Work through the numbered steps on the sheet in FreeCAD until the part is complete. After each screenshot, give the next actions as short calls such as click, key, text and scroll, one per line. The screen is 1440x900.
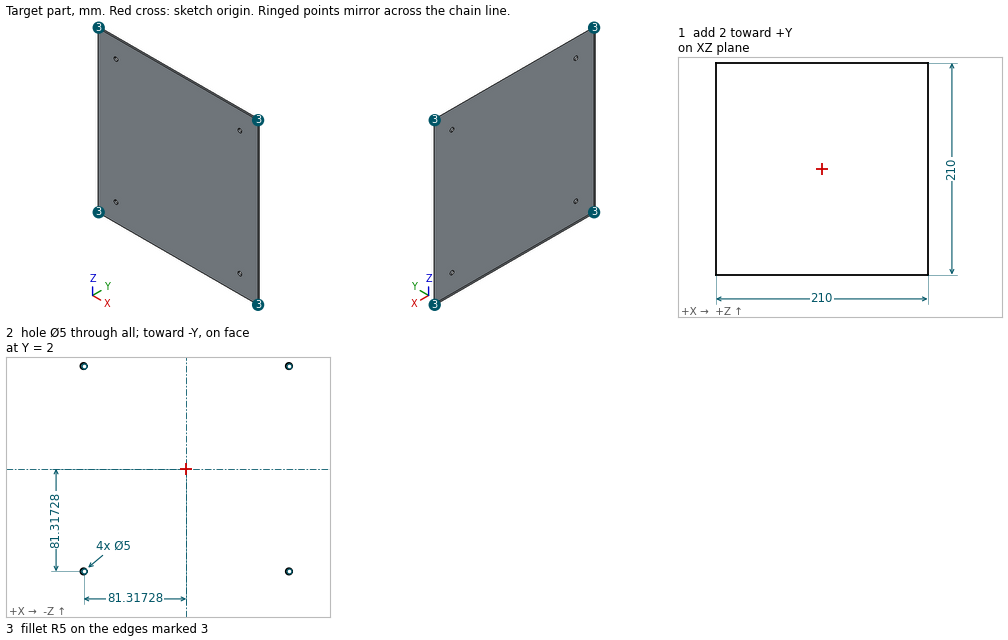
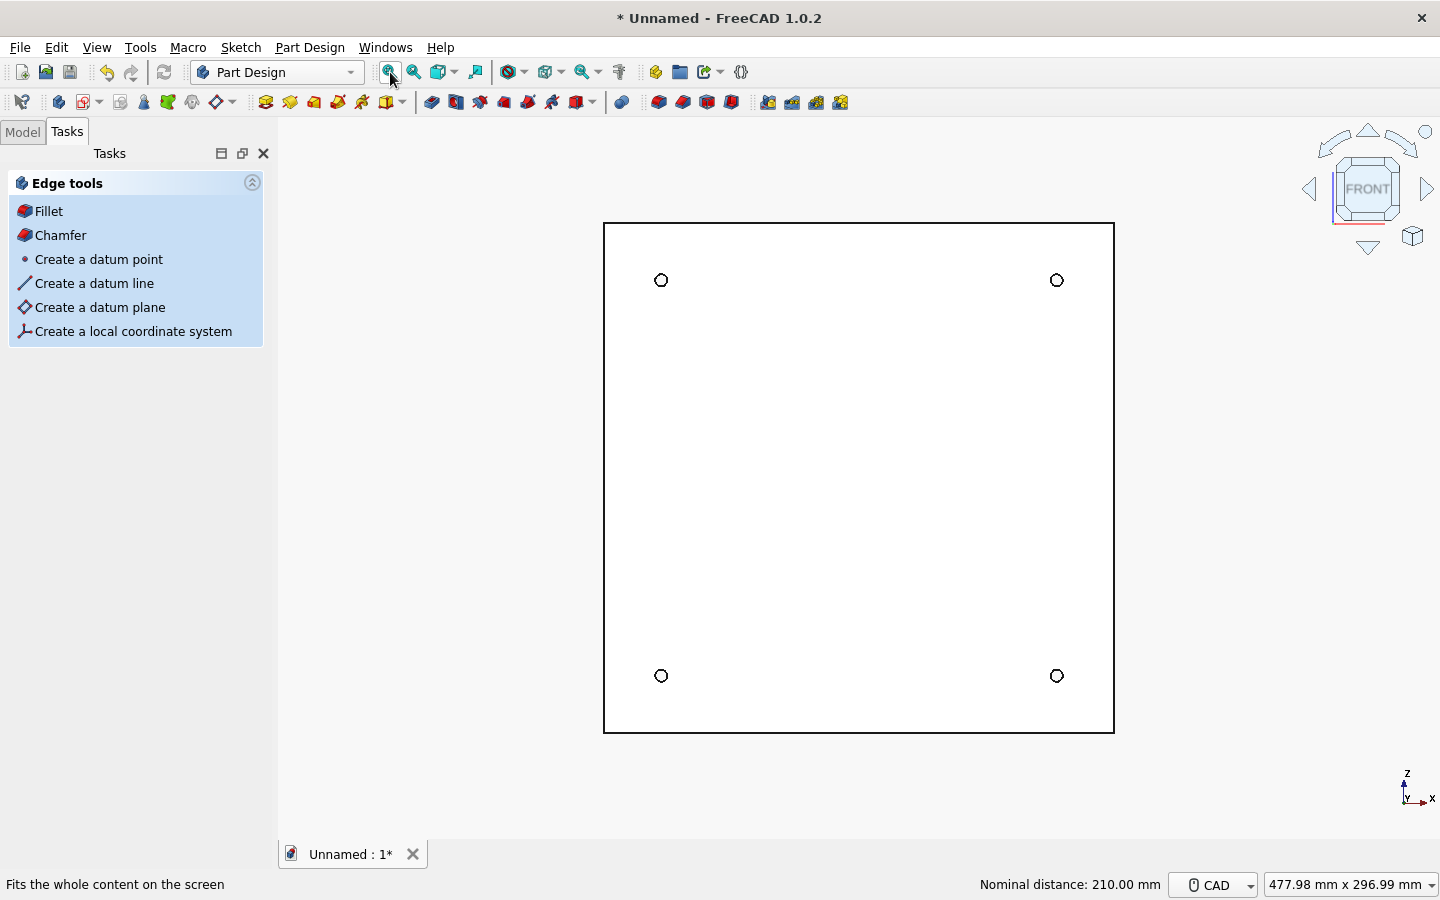
key(3)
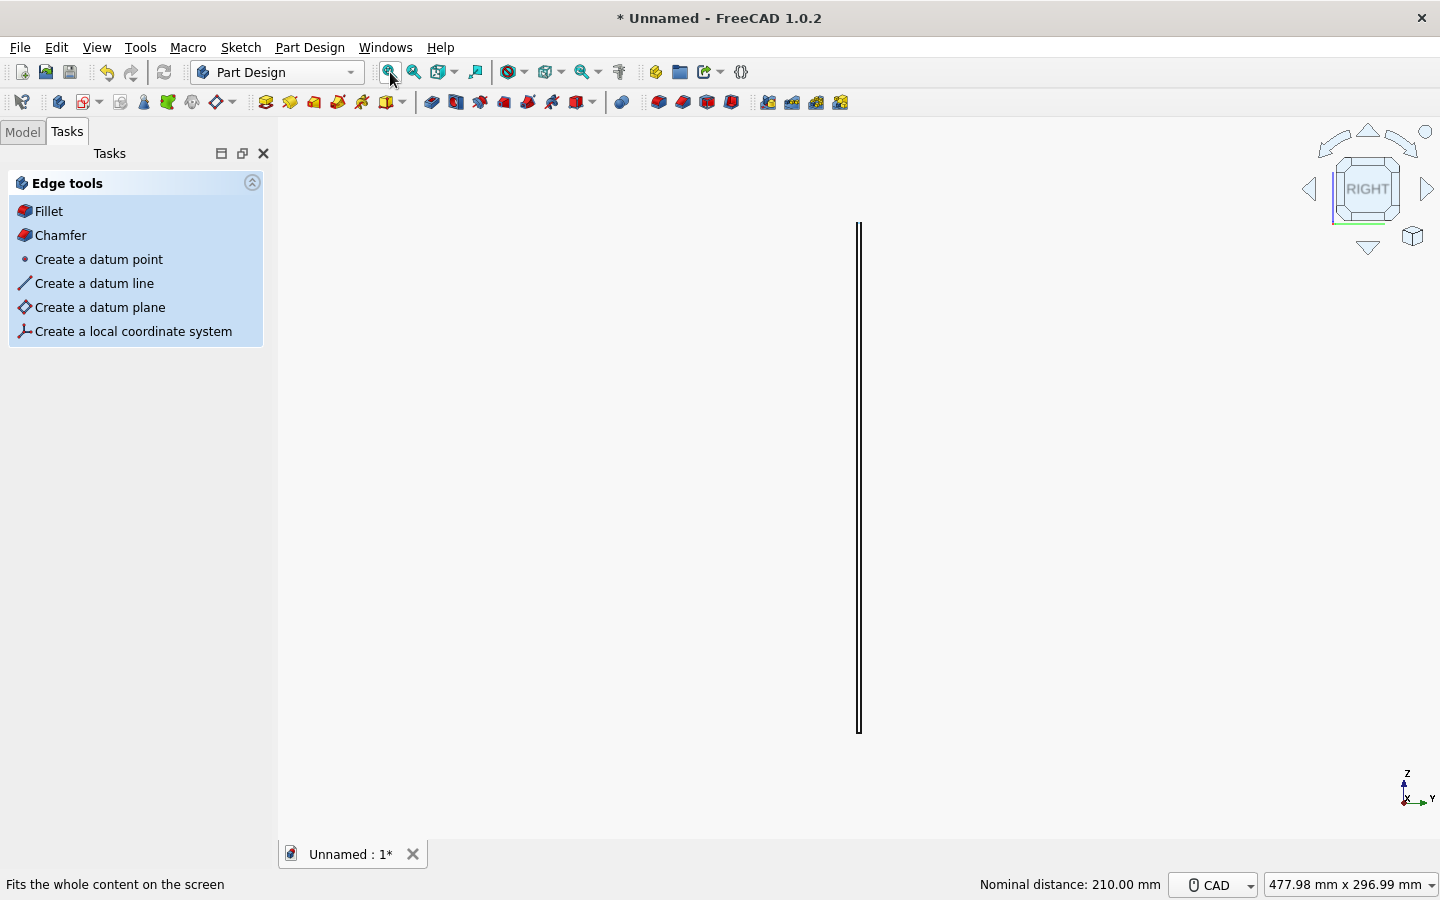
scroll(859, 732, up, 11)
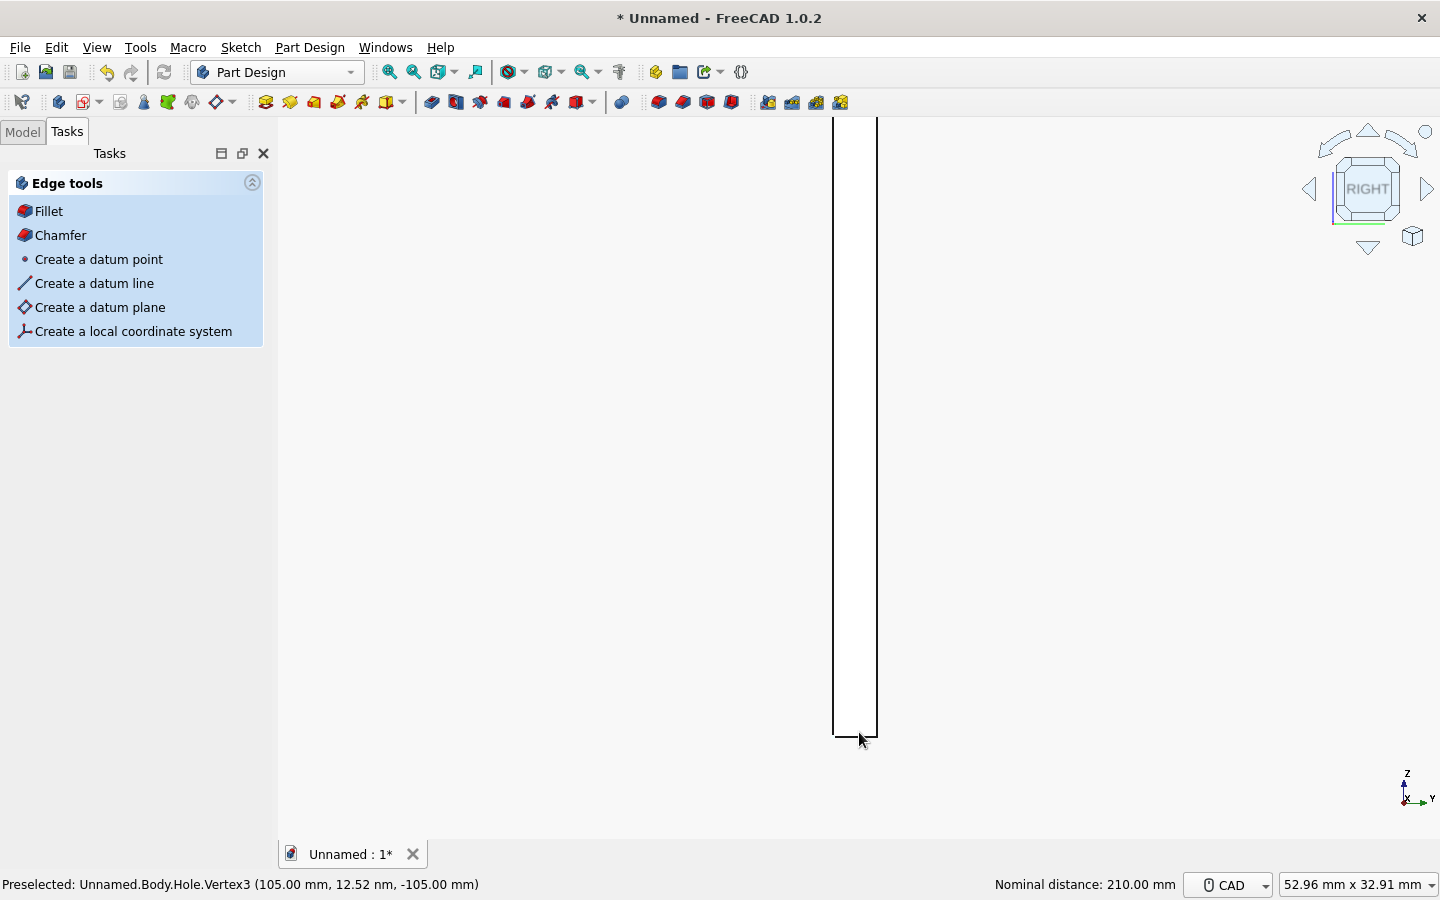
click(855, 736, ctrl)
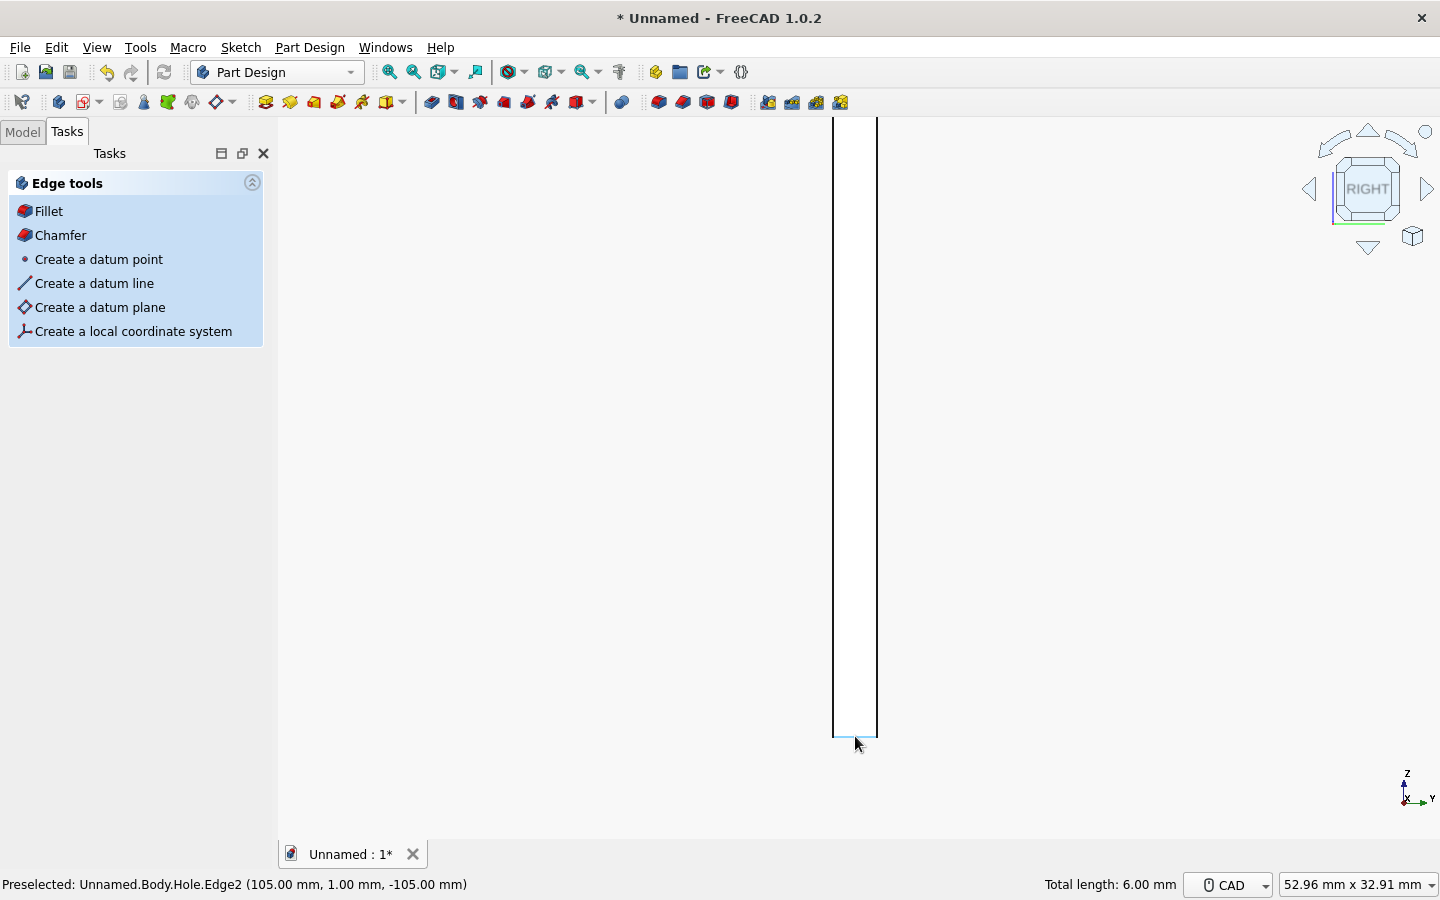
click(390, 72)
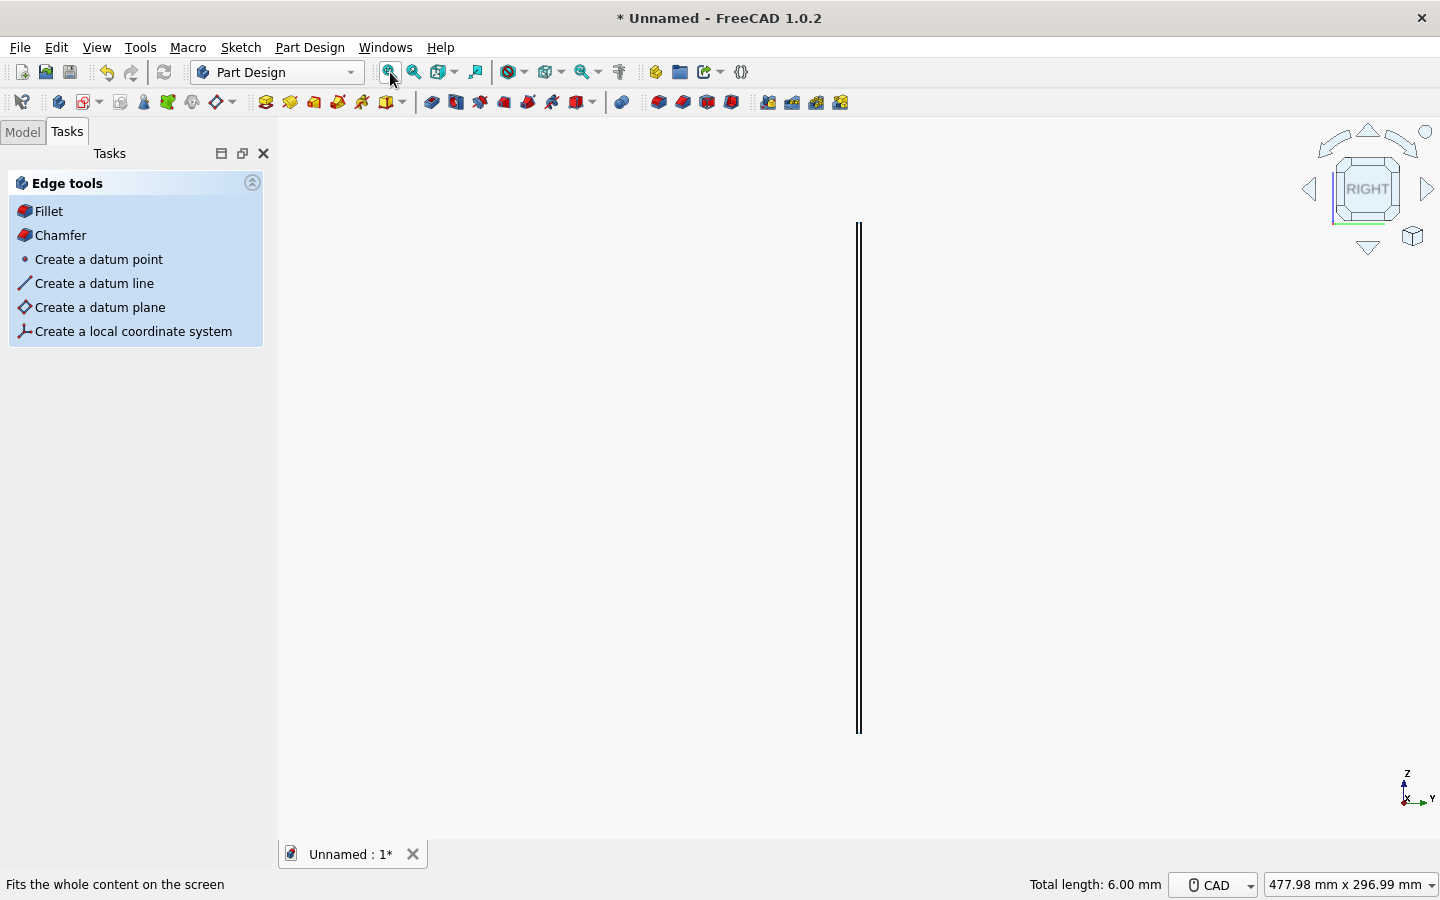
key(5)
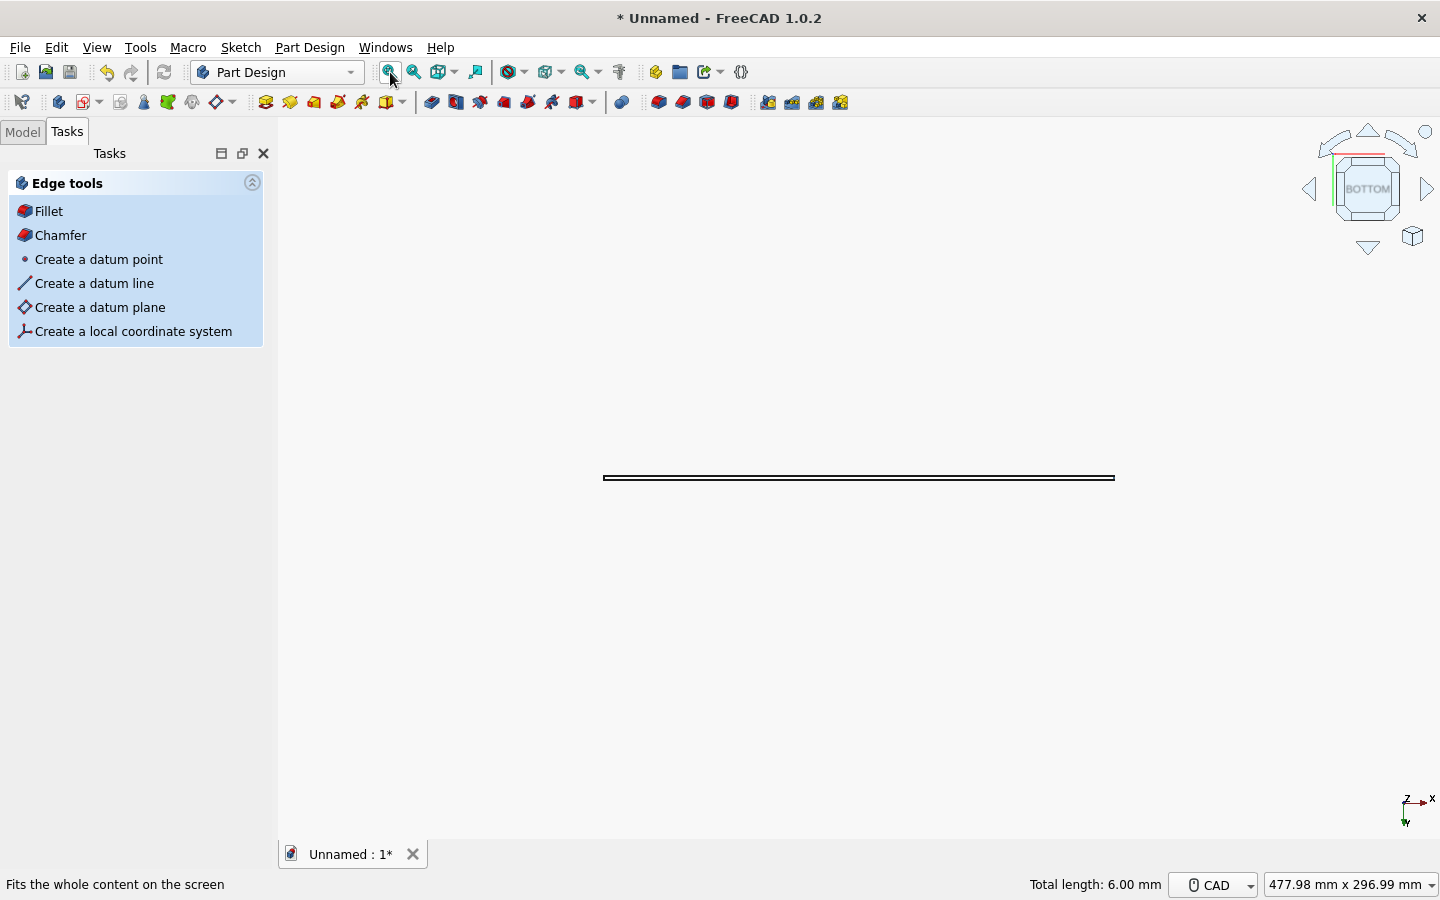
click(390, 72)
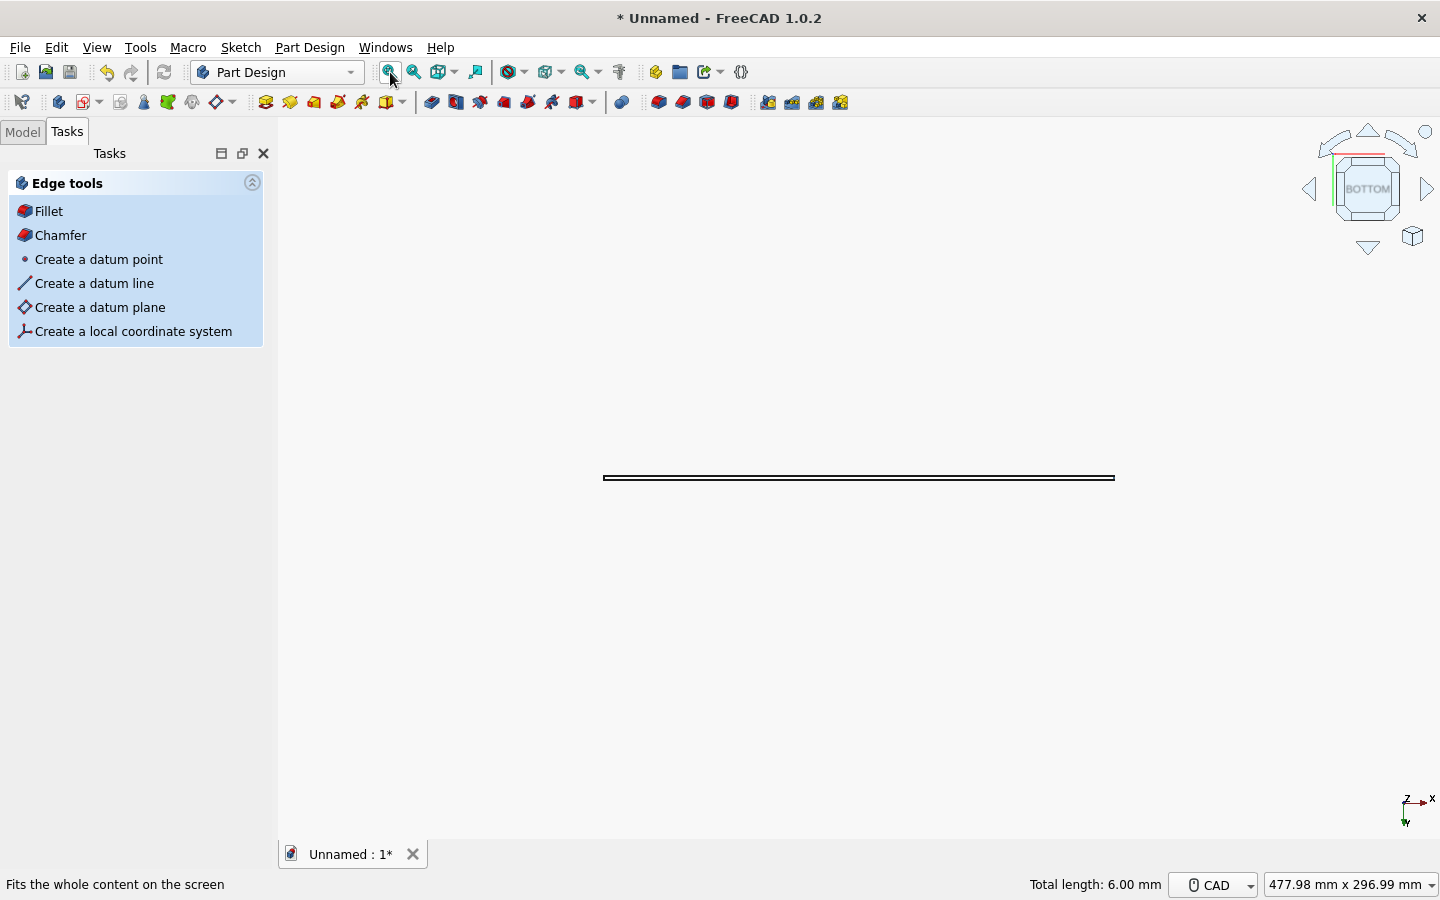
scroll(604, 477, up, 11)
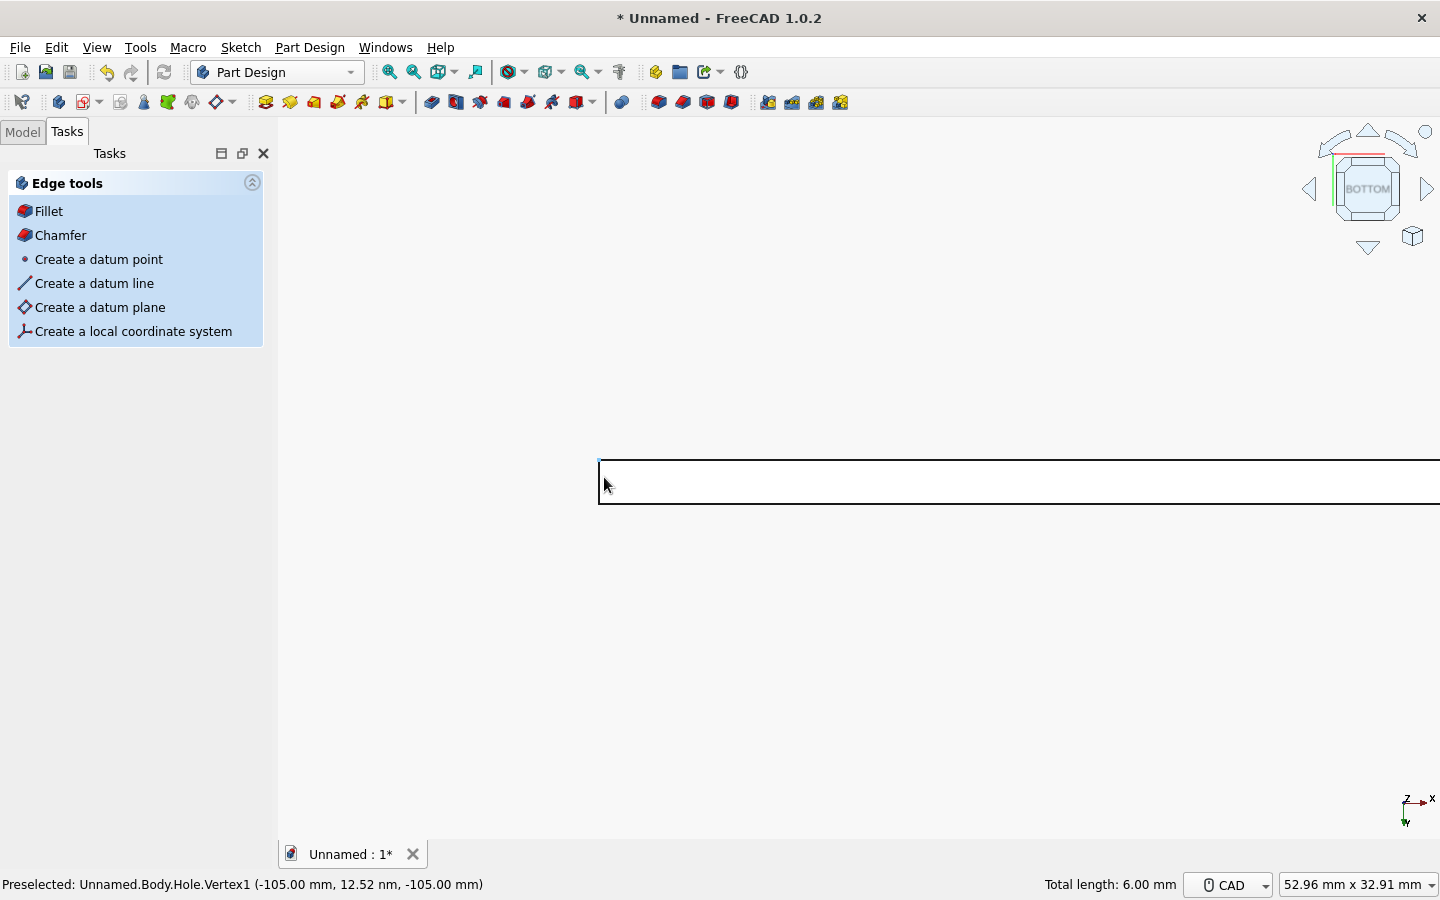
click(599, 481, ctrl)